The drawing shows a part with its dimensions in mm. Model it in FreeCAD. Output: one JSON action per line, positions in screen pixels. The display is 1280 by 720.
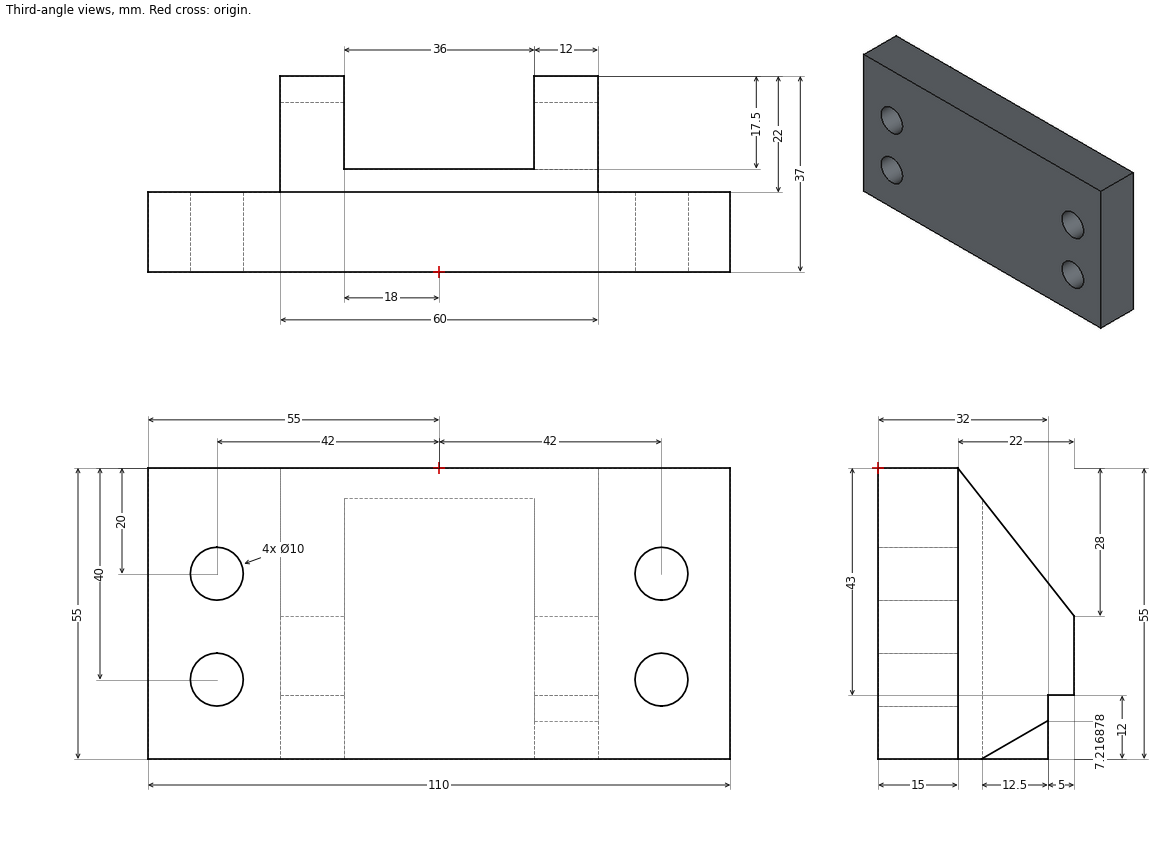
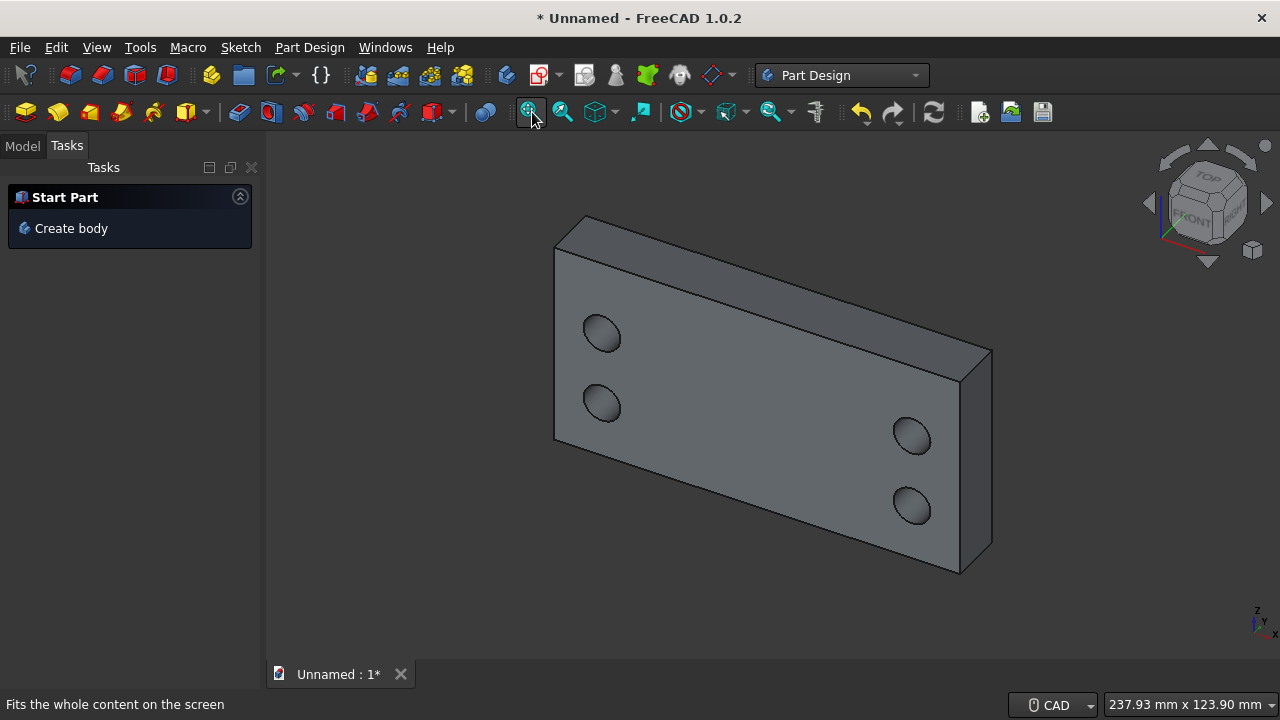
{"action": "key", "text": "5"}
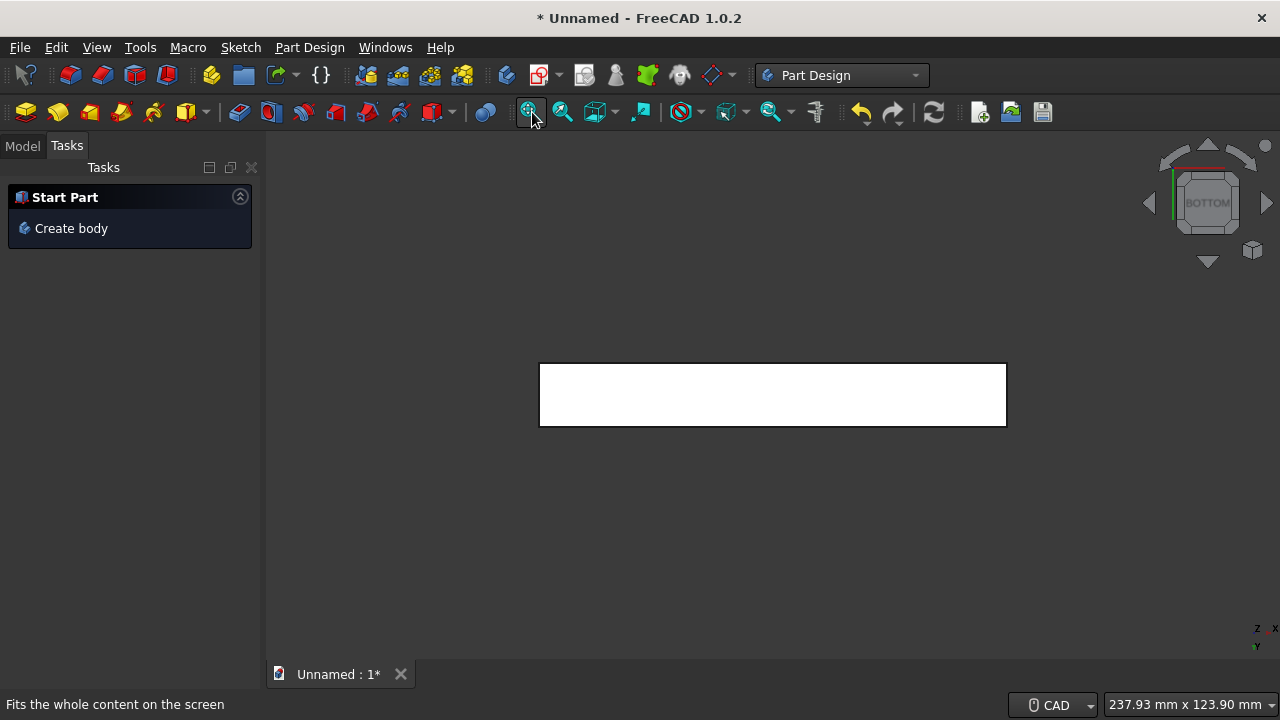
{"action": "left_click", "coordinate": [974, 394]}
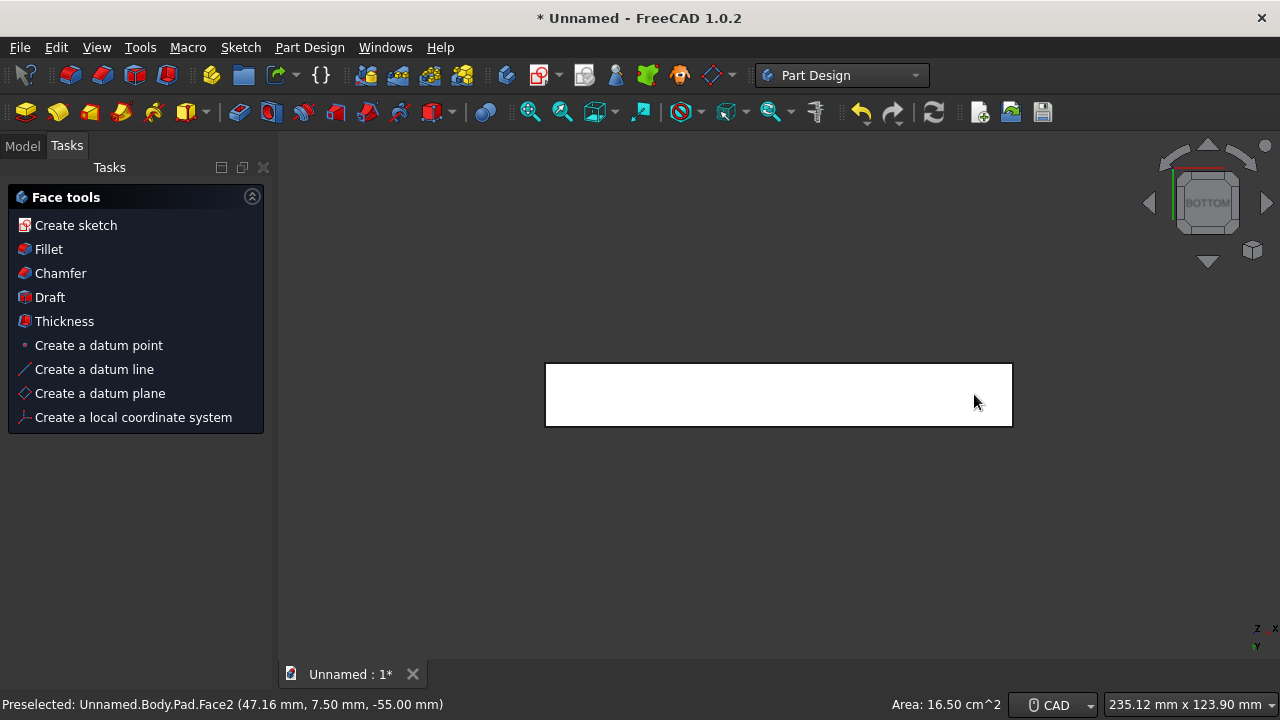
{"action": "left_click", "coordinate": [540, 76]}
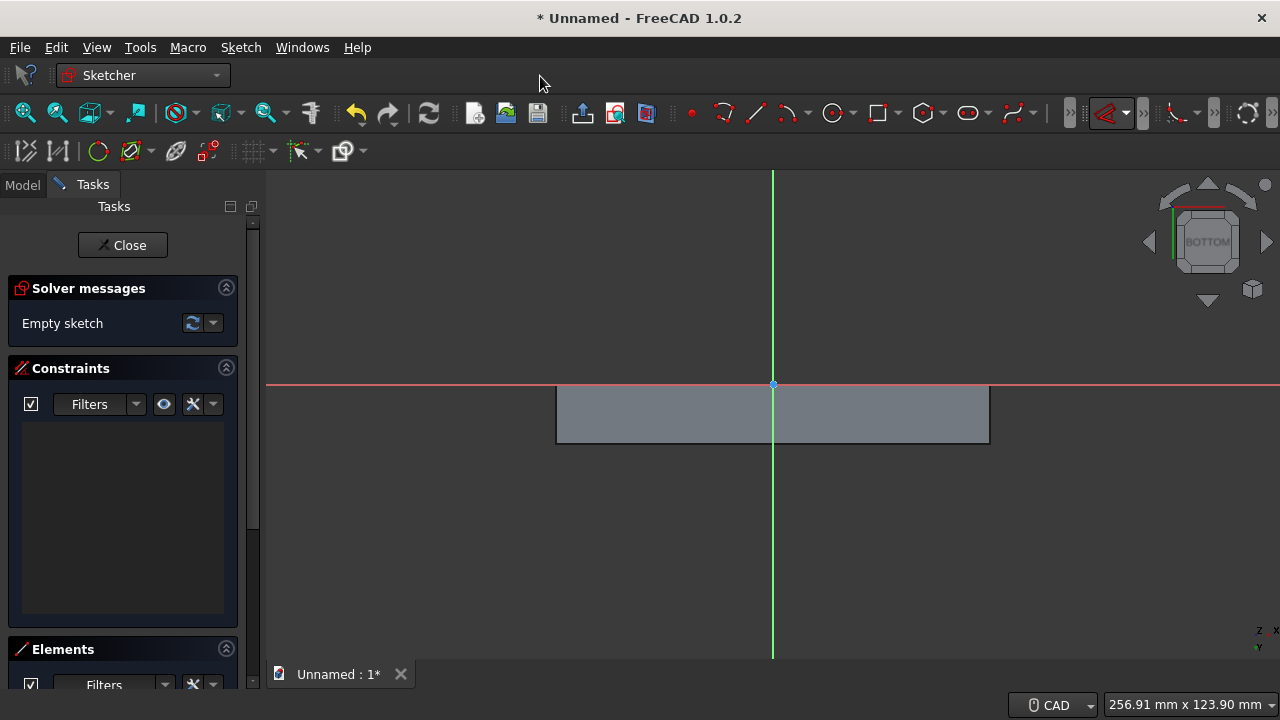
{"action": "scroll", "coordinate": [829, 493], "scroll_direction": "up", "scroll_amount": 4}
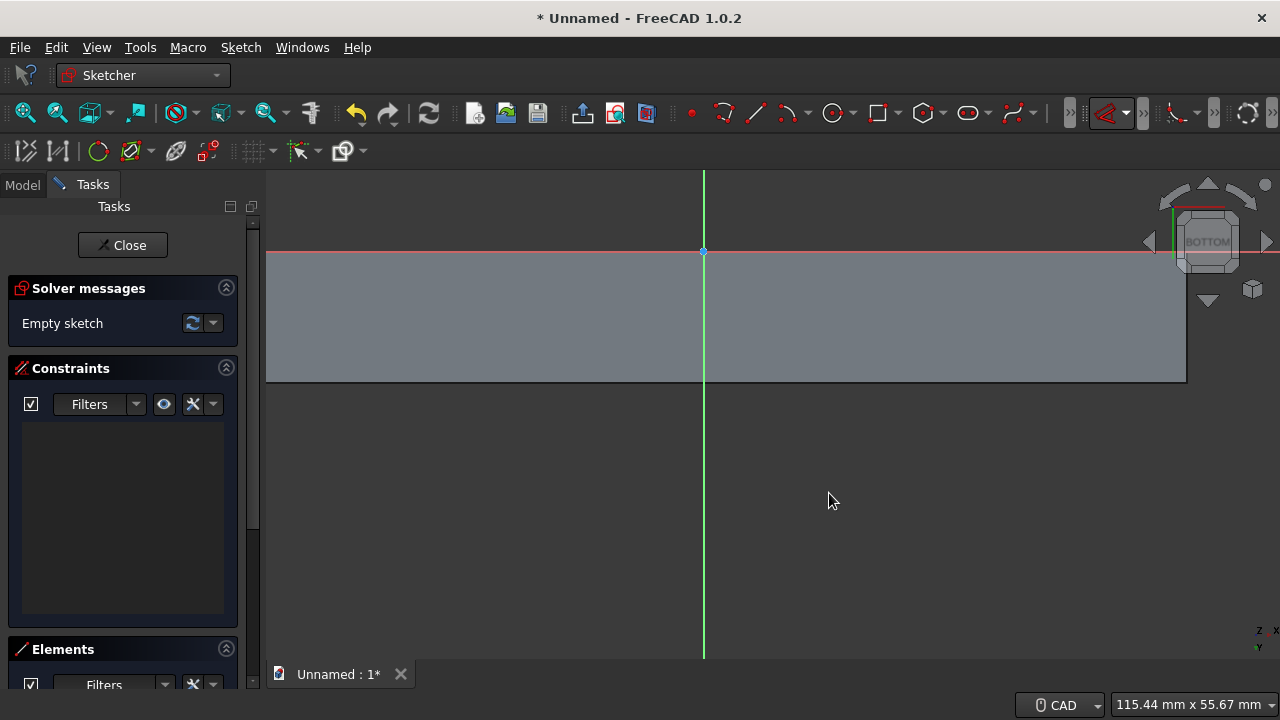
{"action": "left_click", "coordinate": [724, 114]}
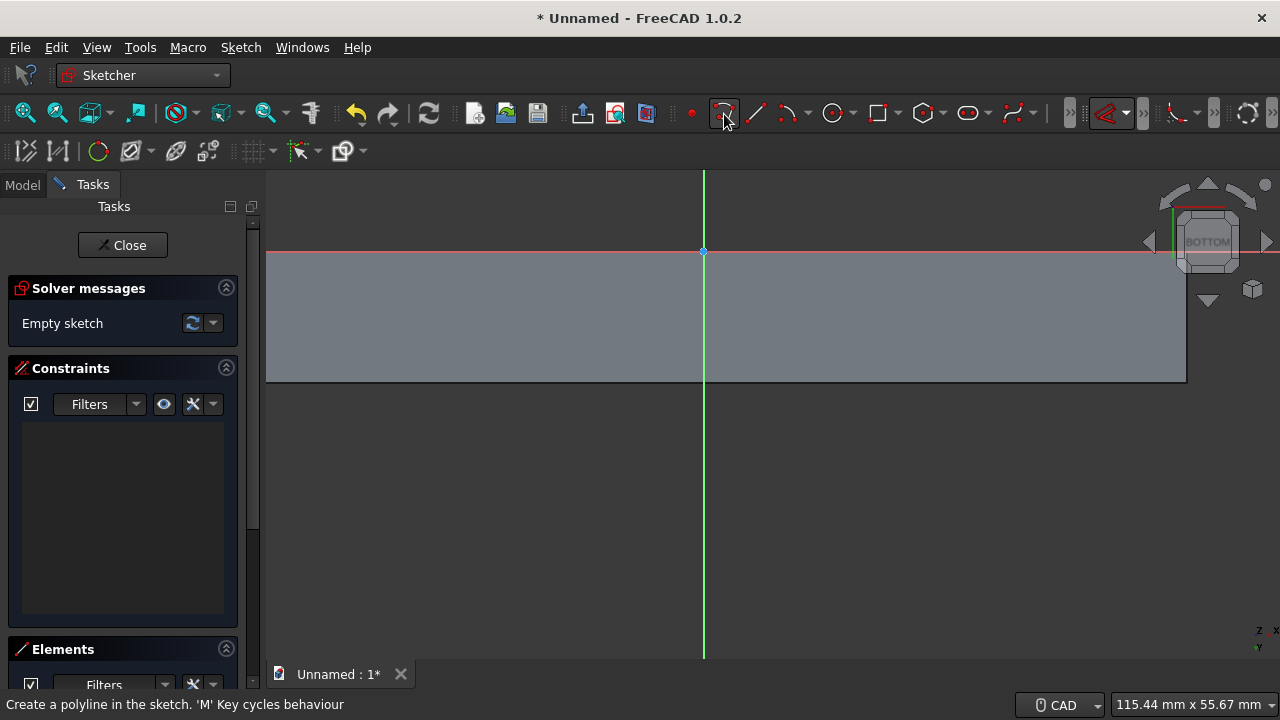
{"action": "left_click", "coordinate": [546, 423]}
{"action": "left_click", "coordinate": [862, 423]}
{"action": "left_click", "coordinate": [862, 577]}
{"action": "left_click", "coordinate": [967, 577]}
{"action": "left_click", "coordinate": [967, 383]}
{"action": "left_click", "coordinate": [440, 383]}
{"action": "left_click", "coordinate": [440, 577]}
{"action": "left_click", "coordinate": [546, 577]}
{"action": "left_click", "coordinate": [546, 424]}
{"action": "key", "text": "Escape"}
{"action": "key", "text": "Escape"}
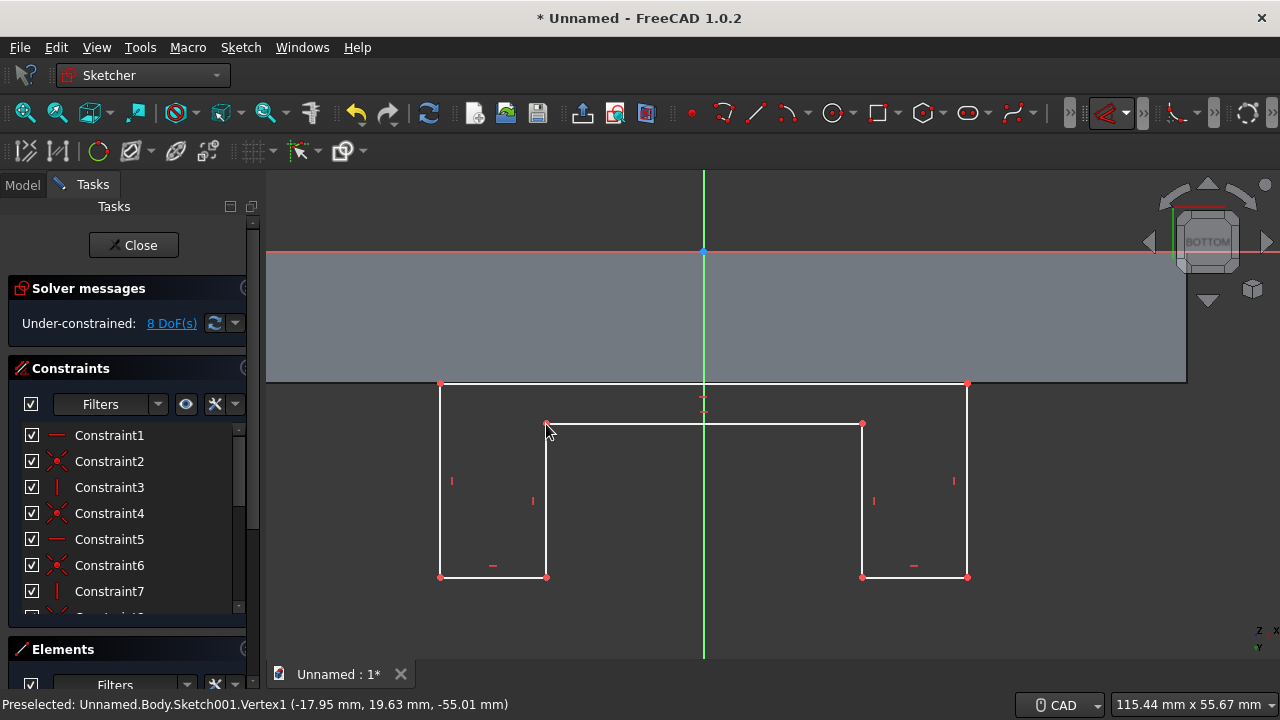
{"action": "left_click", "coordinate": [641, 424]}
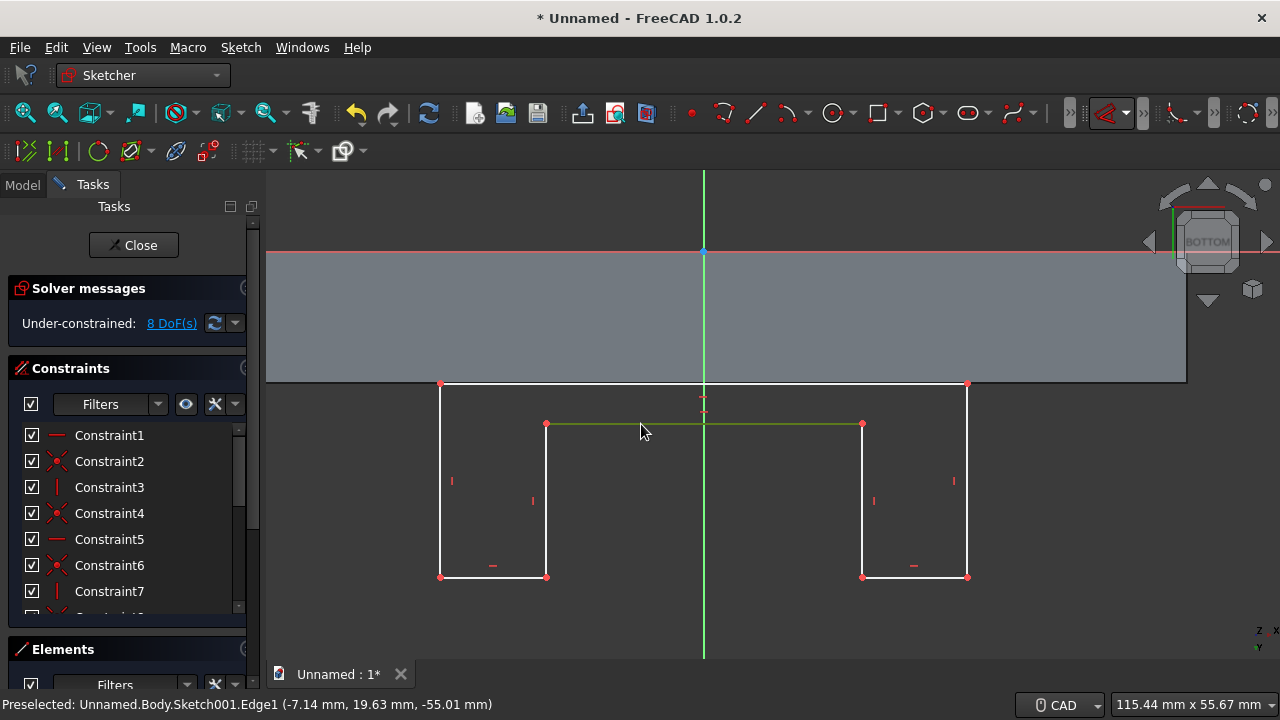
{"action": "left_click", "coordinate": [1128, 114]}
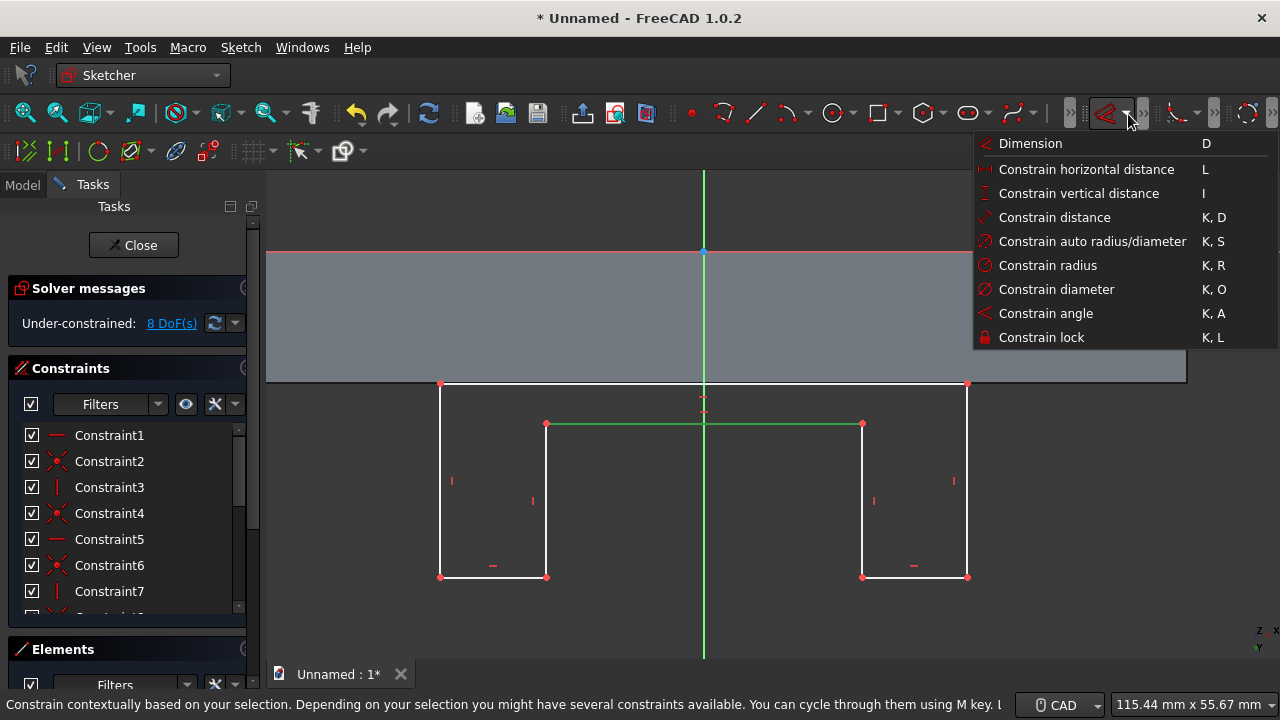
{"action": "left_click", "coordinate": [1126, 169]}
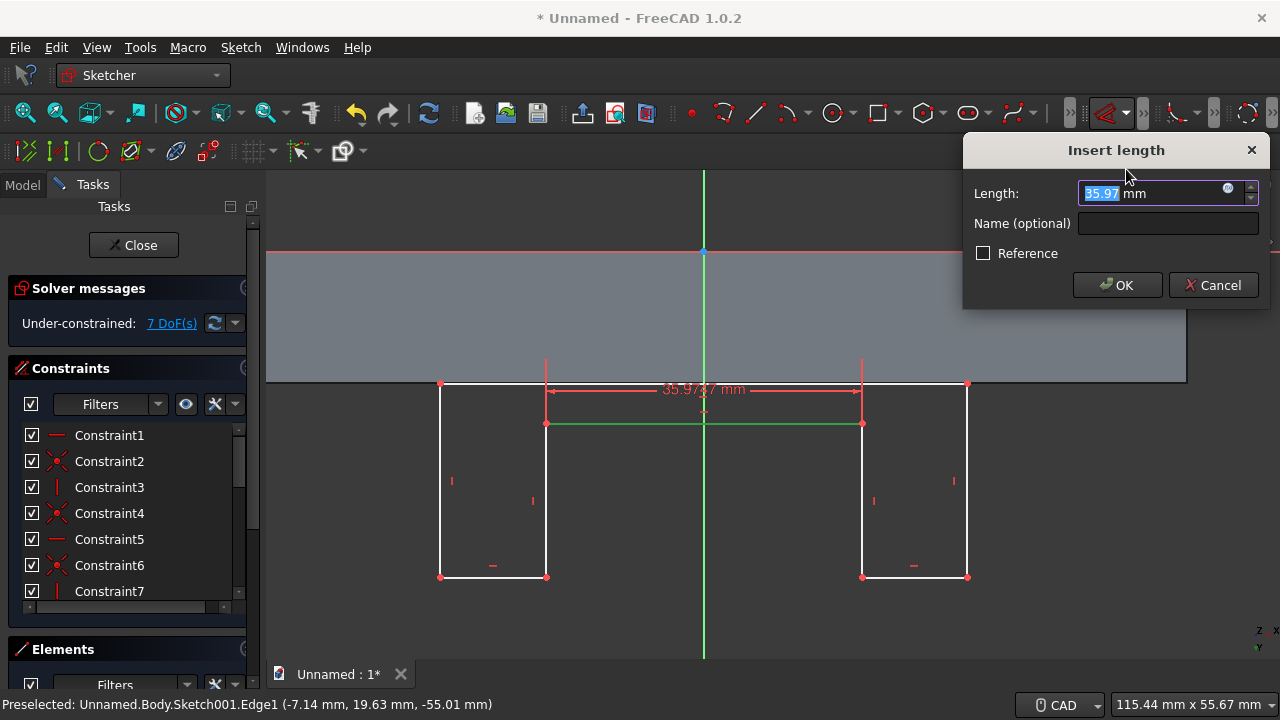
{"action": "type", "text": "36"}
{"action": "key", "text": "Return"}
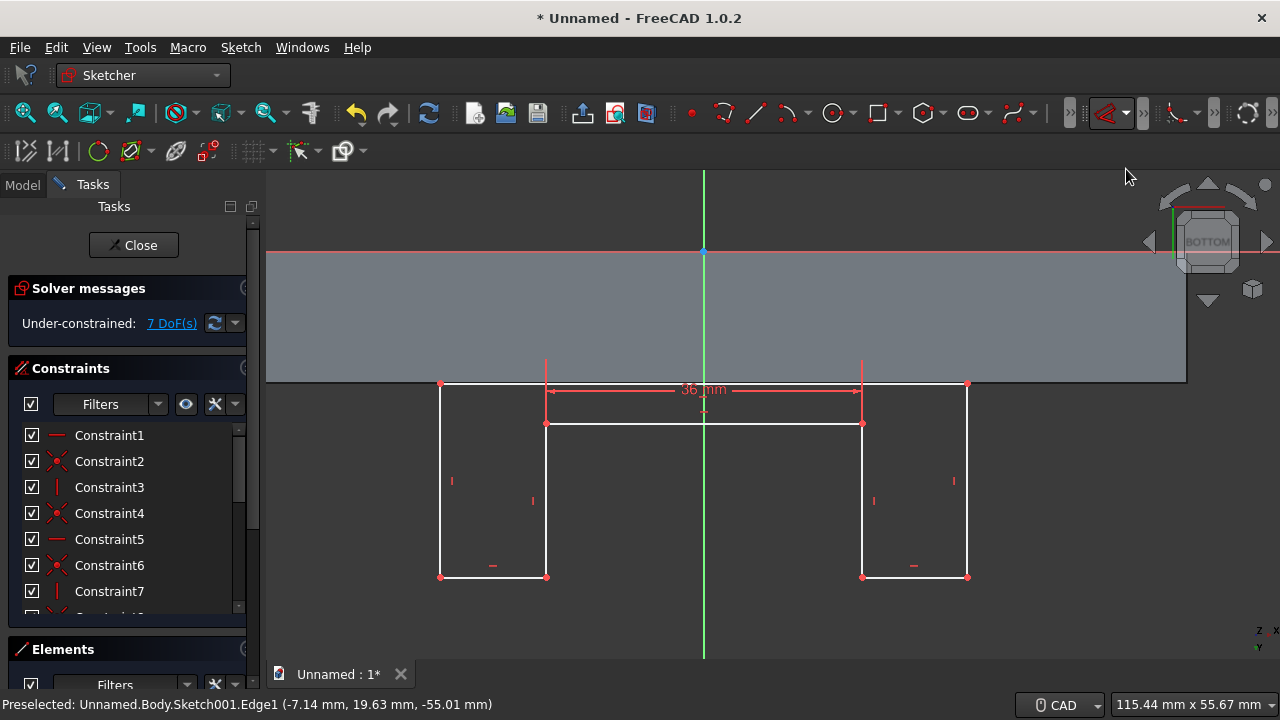
{"action": "left_click", "coordinate": [894, 578]}